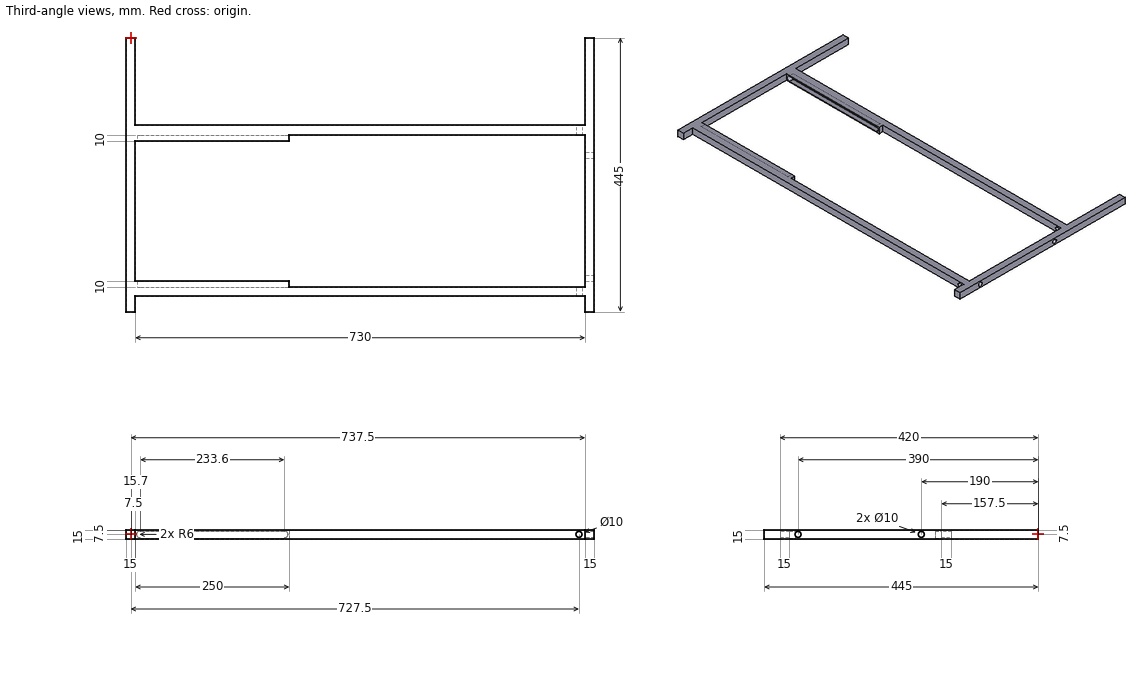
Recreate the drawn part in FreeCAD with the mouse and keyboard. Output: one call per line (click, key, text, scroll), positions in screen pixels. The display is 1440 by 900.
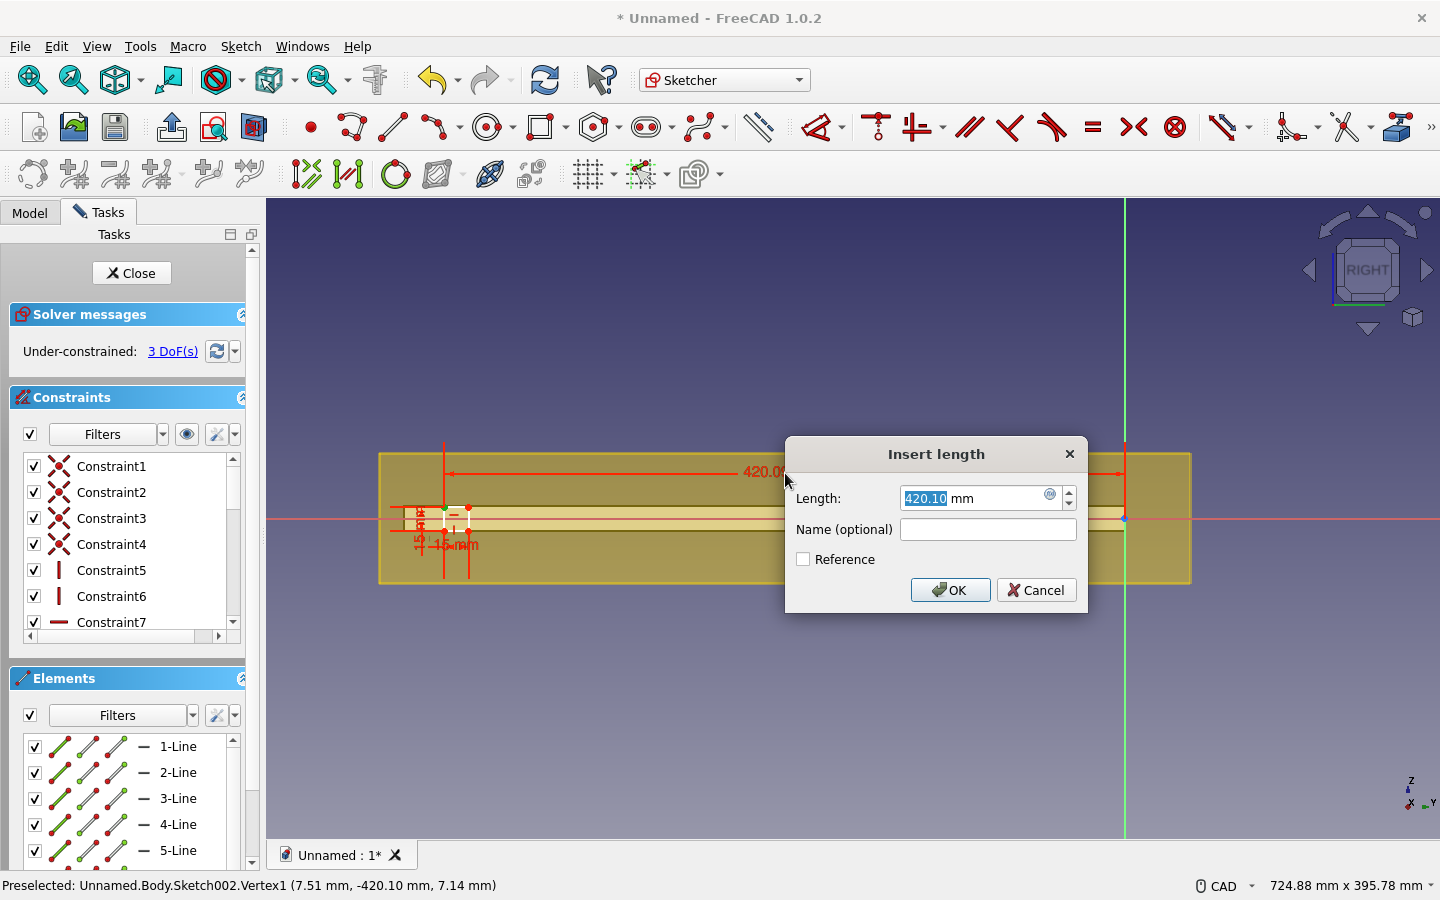
text(420)
key(Return)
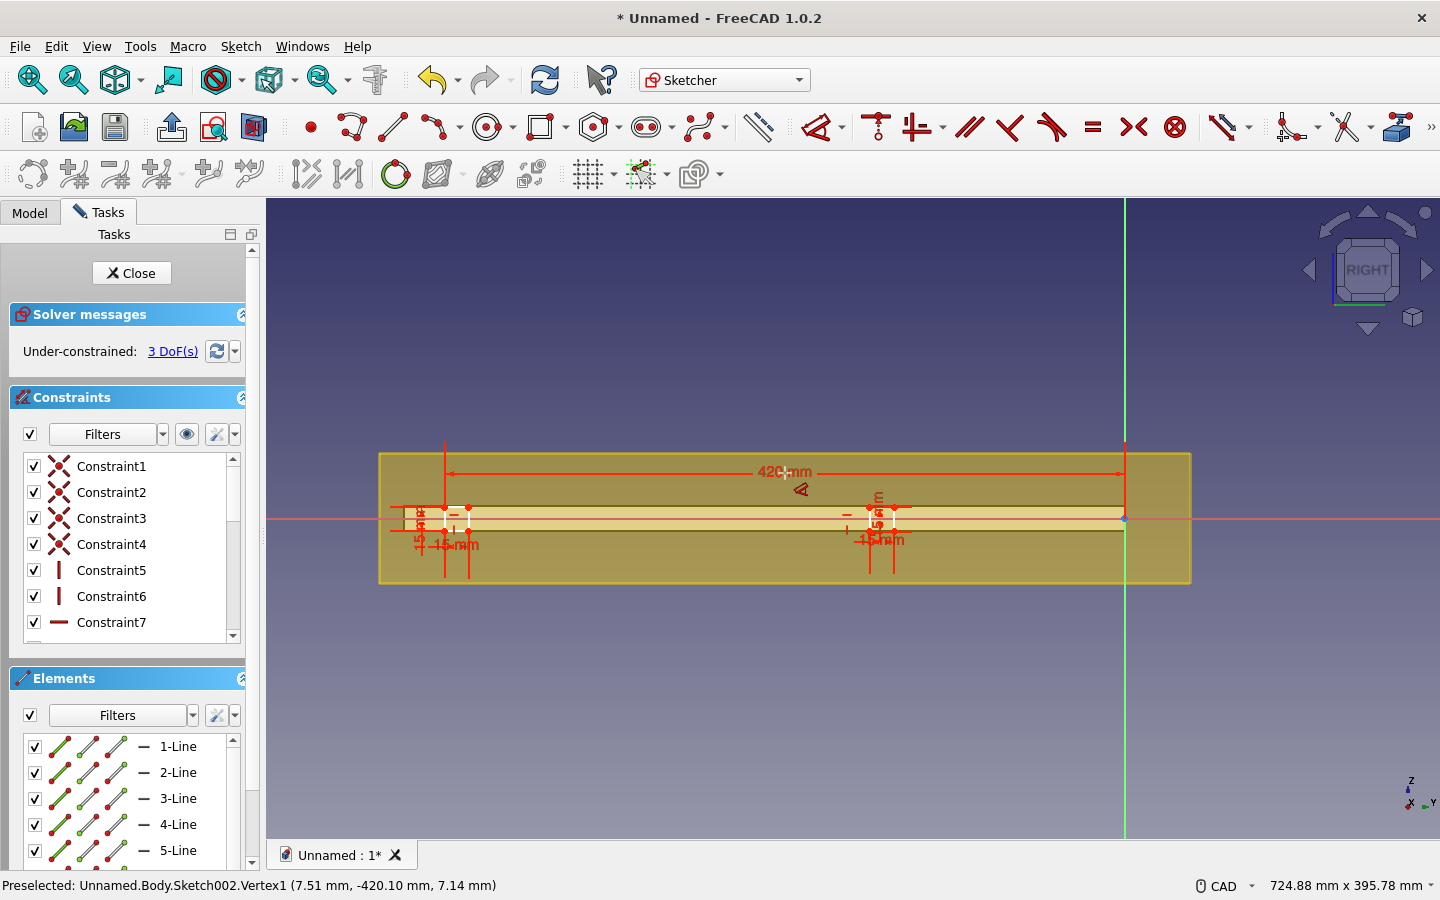
scroll(445, 507, up, 6)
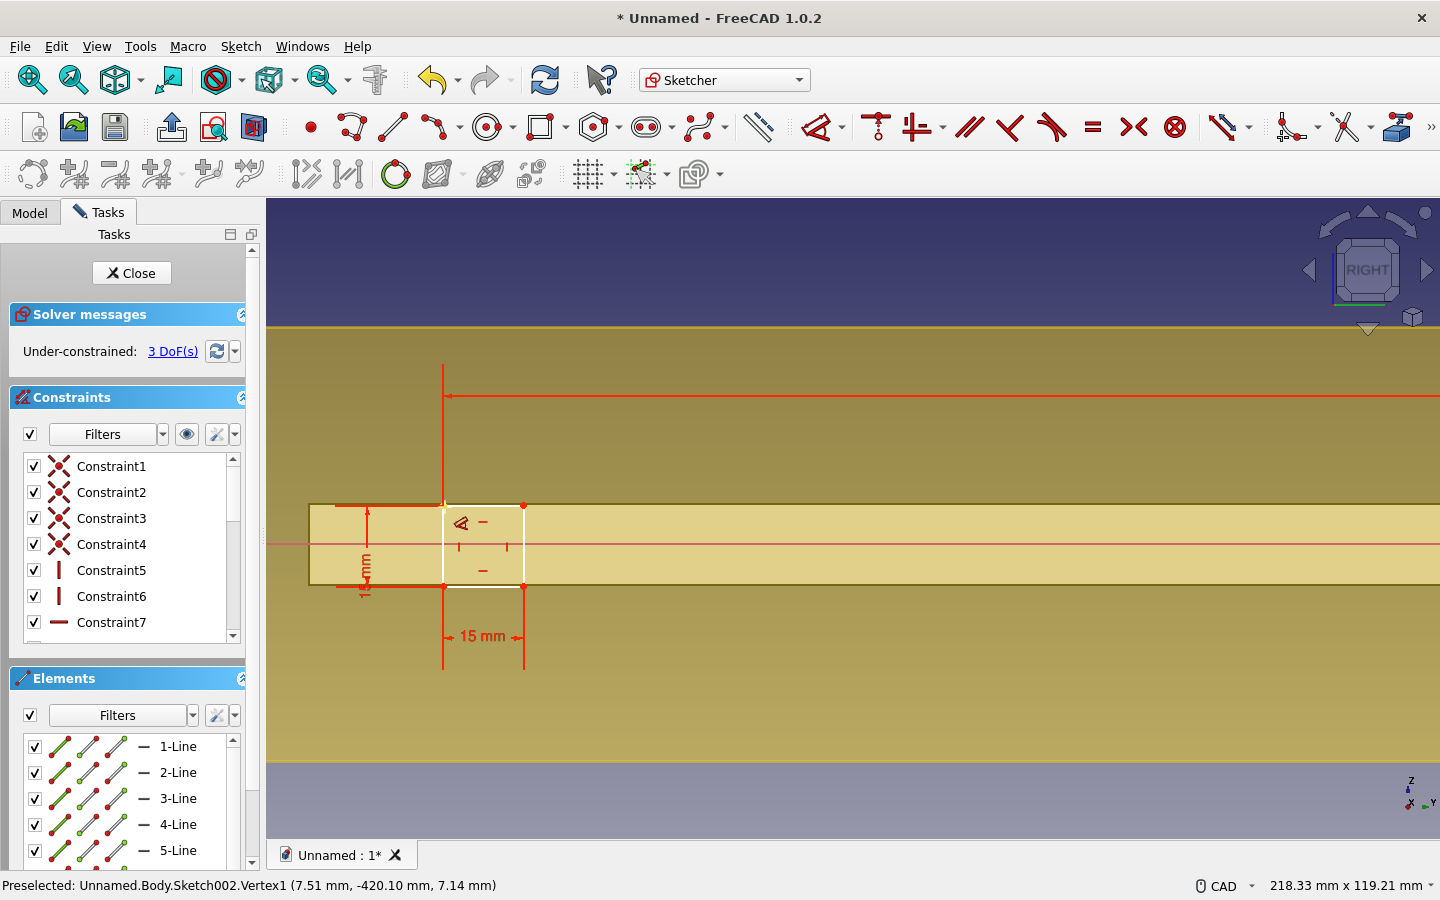
click(443, 506)
click(409, 525)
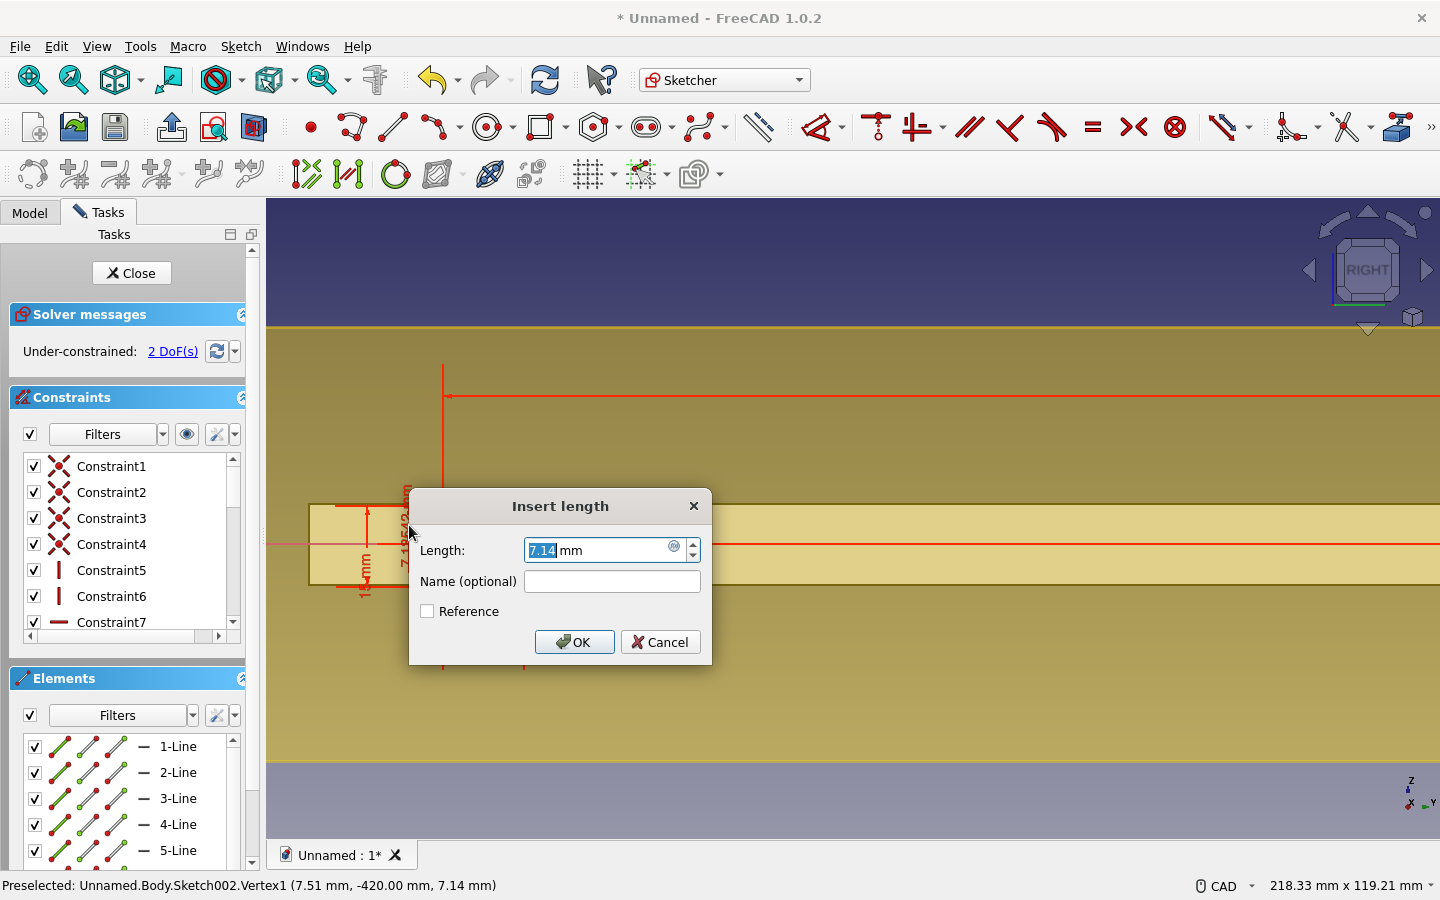
text(7.5)
key(Return)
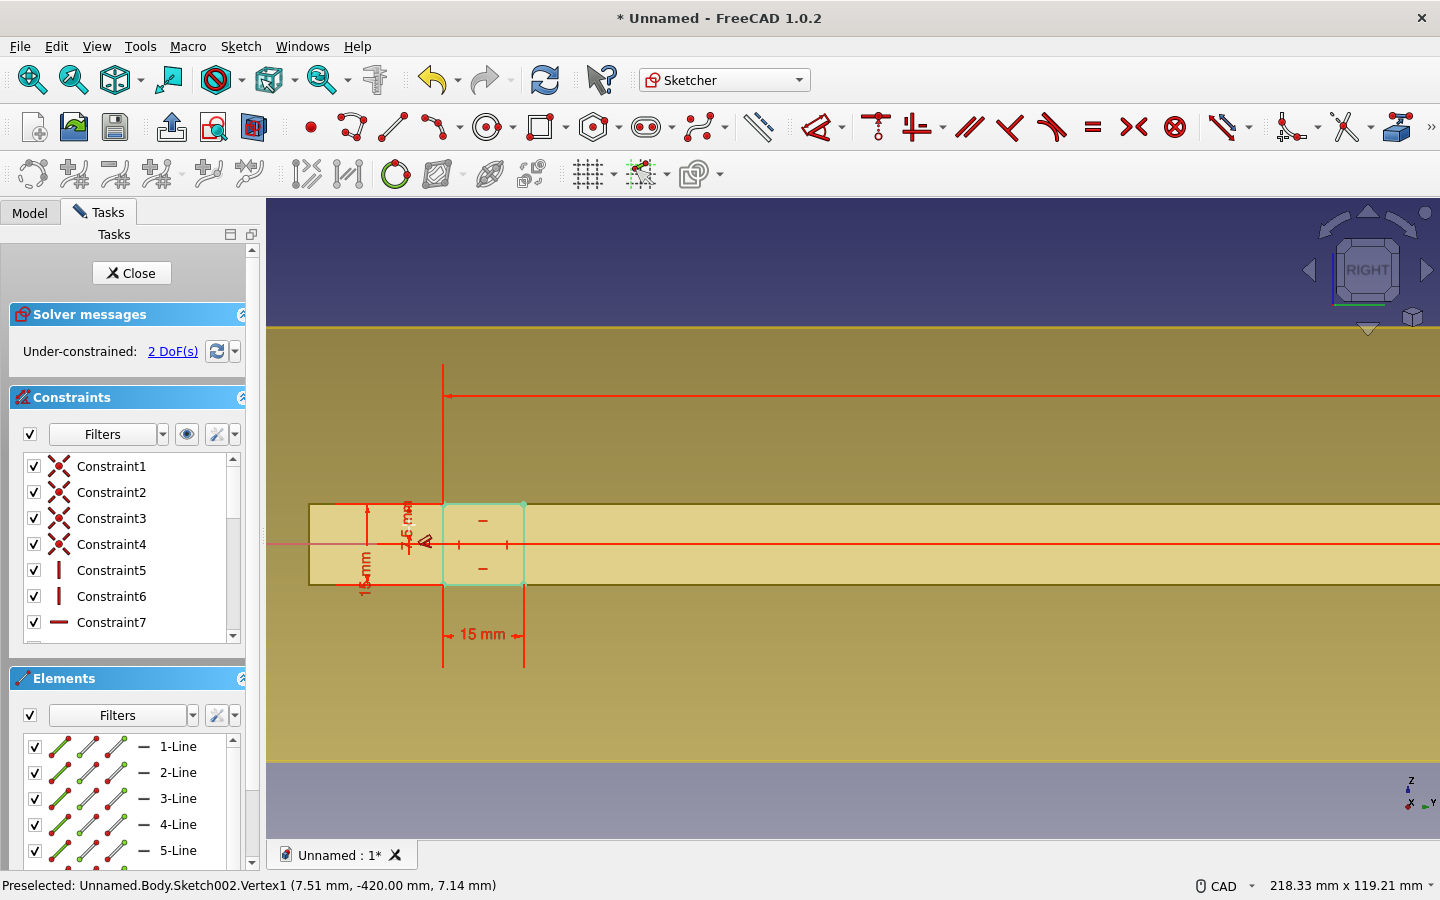
scroll(445, 507, down, 6)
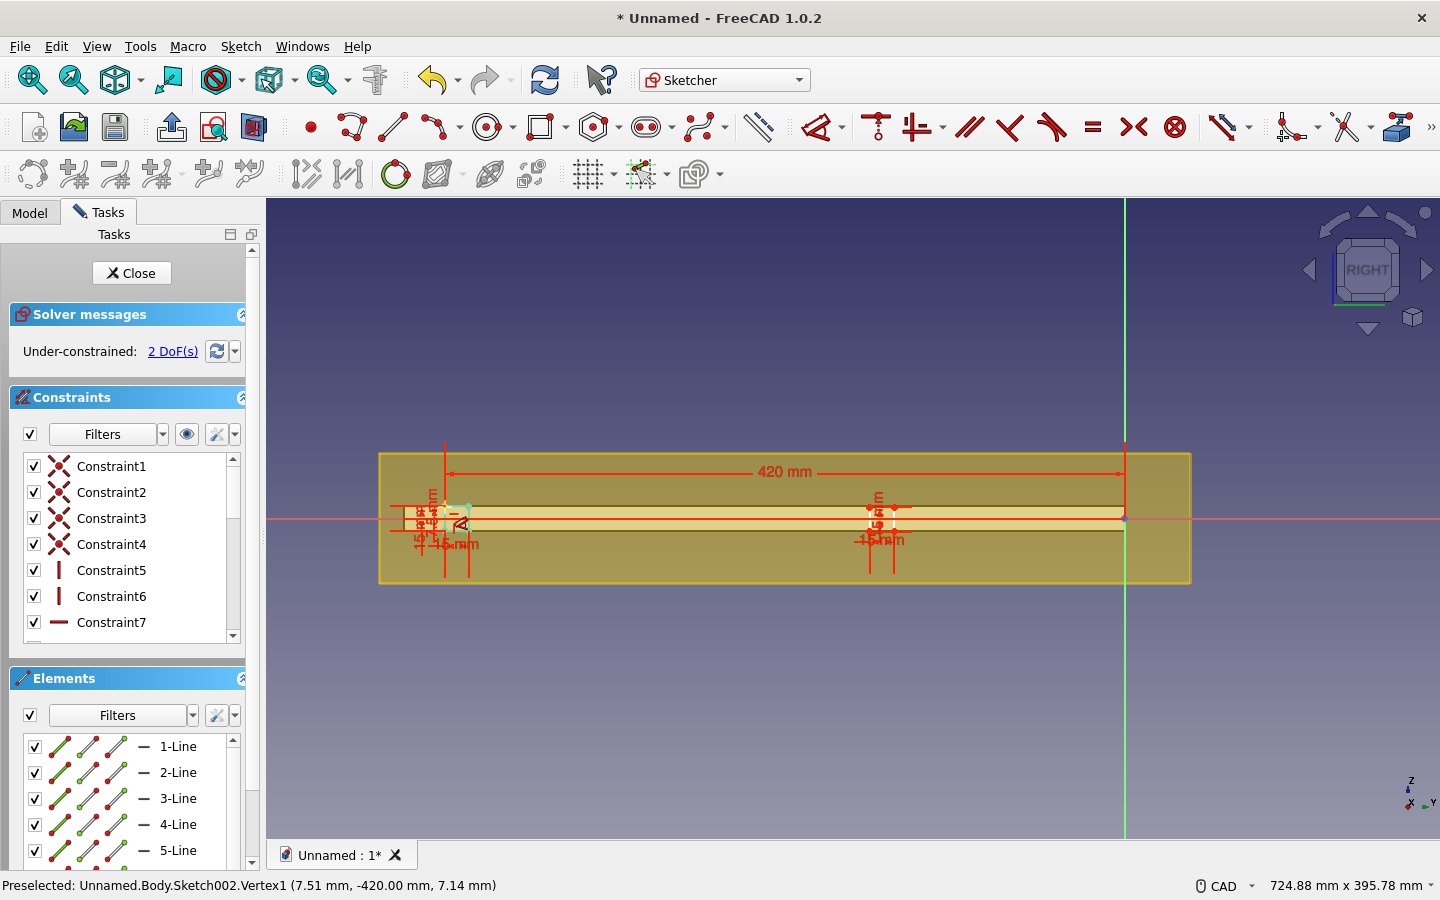
scroll(870, 507, up, 6)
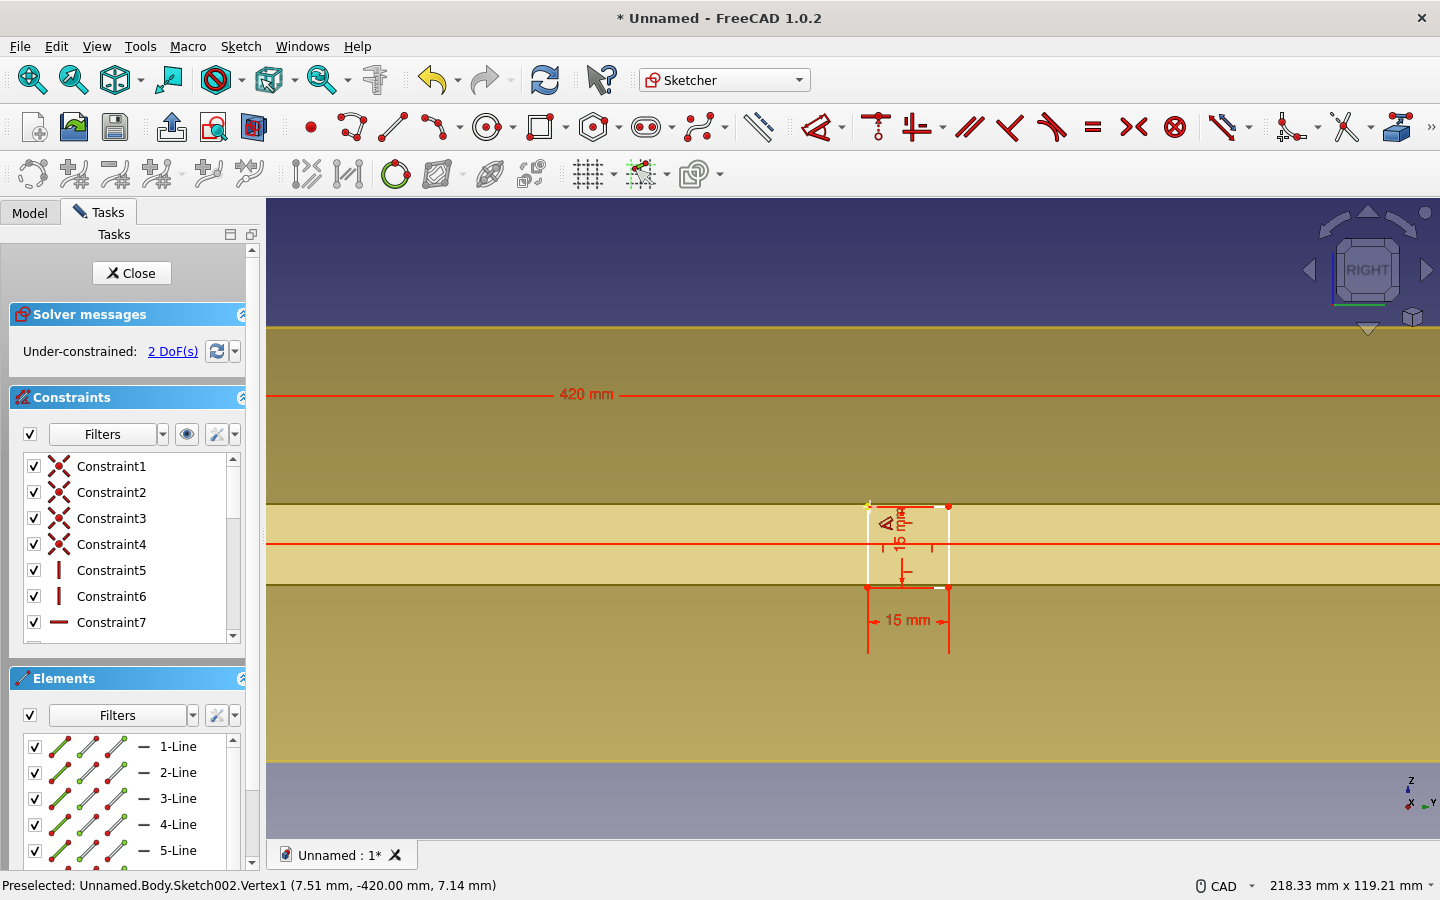
click(868, 507)
click(810, 526)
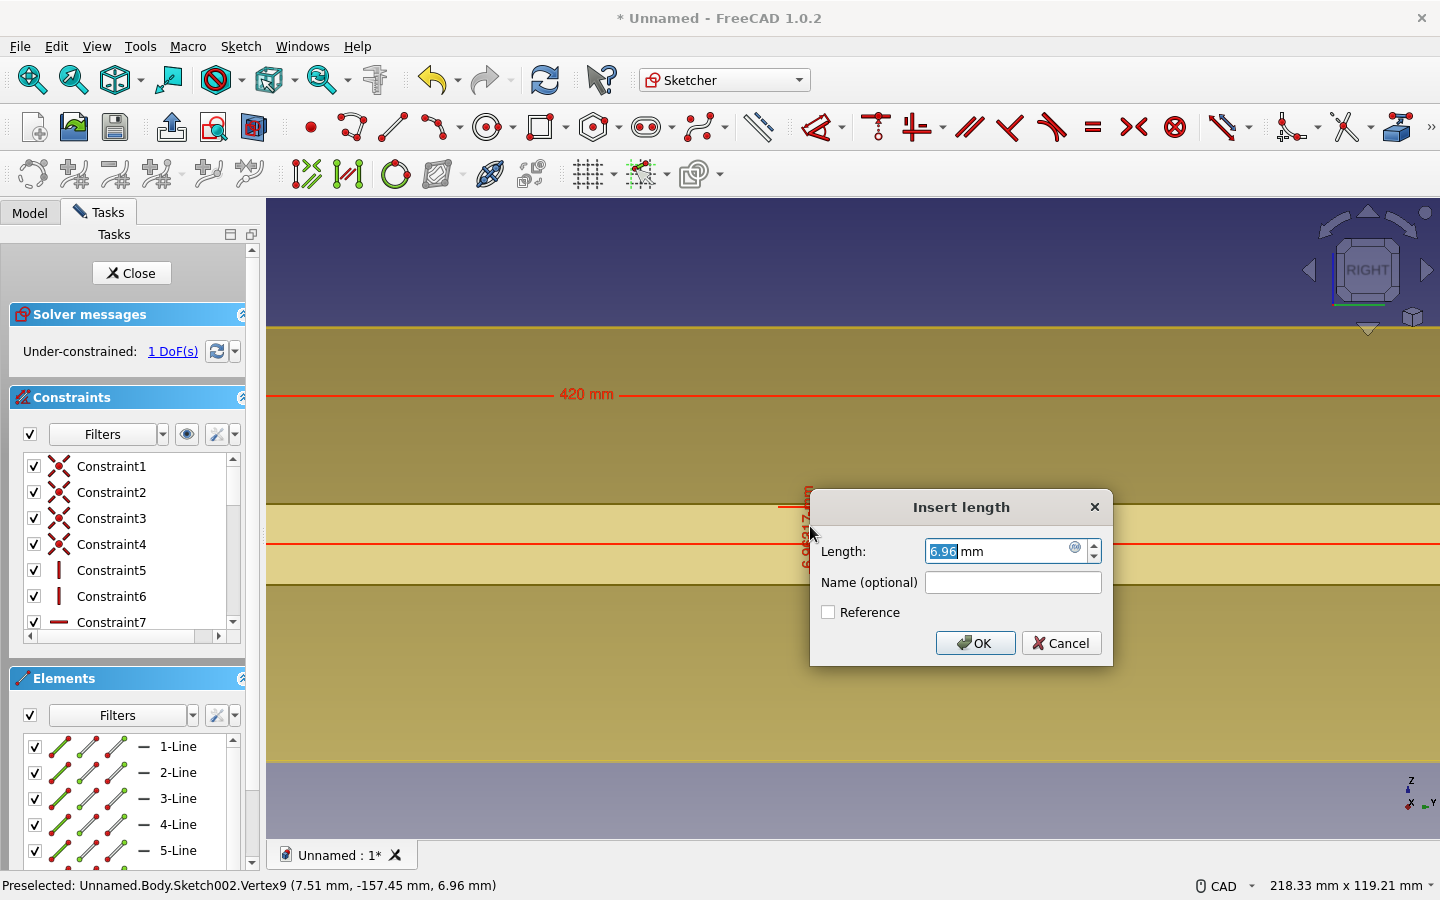
text(7.5)
key(Return)